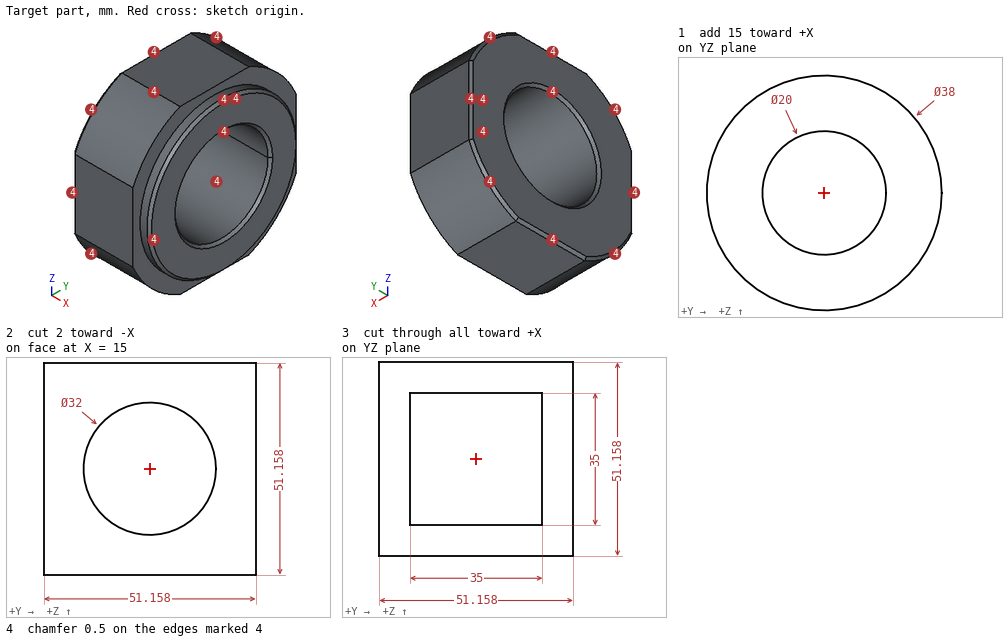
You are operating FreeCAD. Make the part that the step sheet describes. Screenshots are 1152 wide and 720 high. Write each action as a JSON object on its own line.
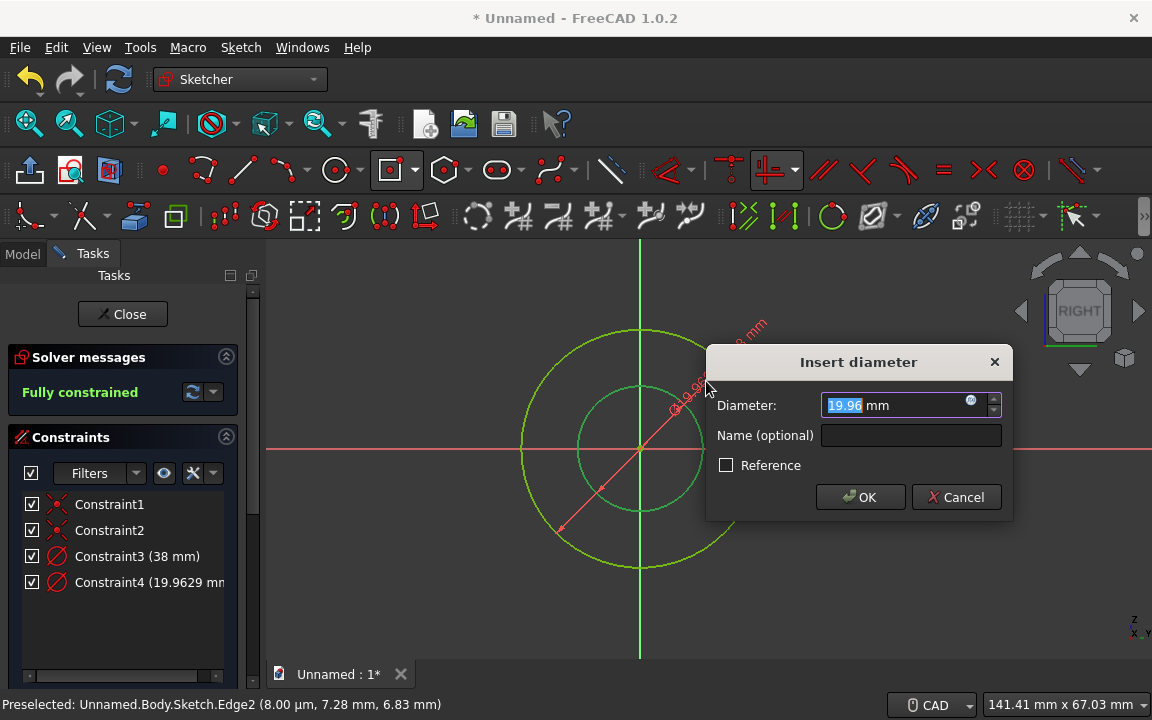
{"action": "type", "text": "20"}
{"action": "key", "text": "Return"}
{"action": "key", "text": "Escape"}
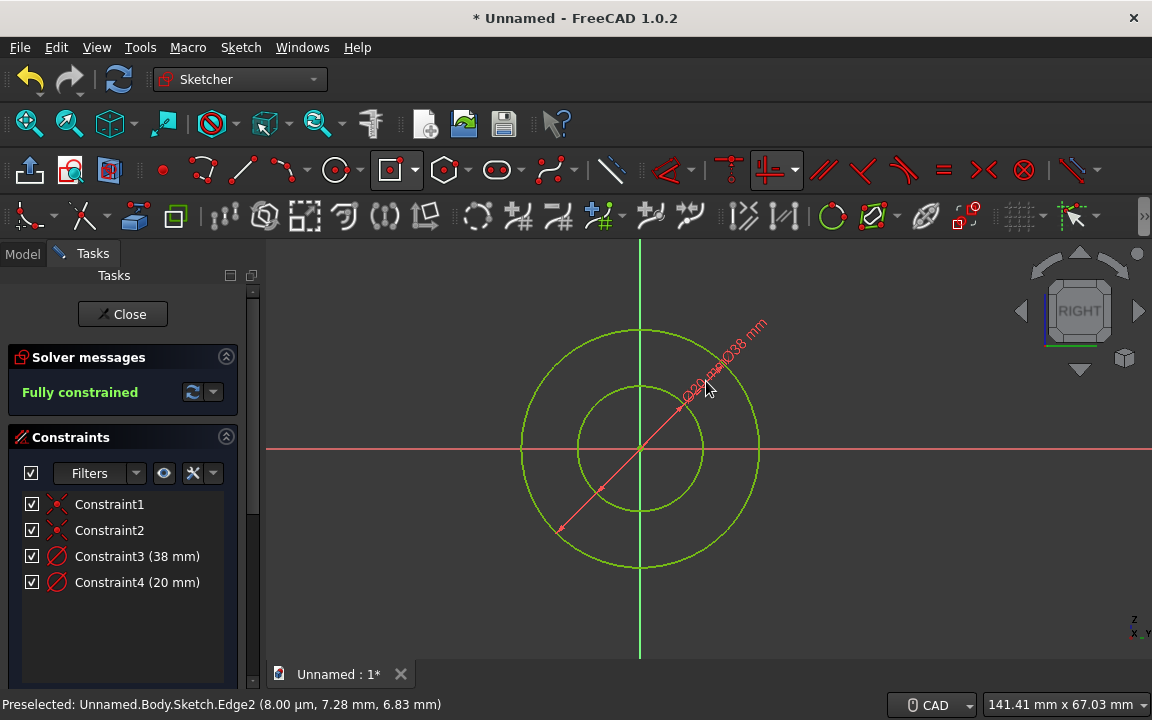
{"action": "left_click", "coordinate": [123, 314]}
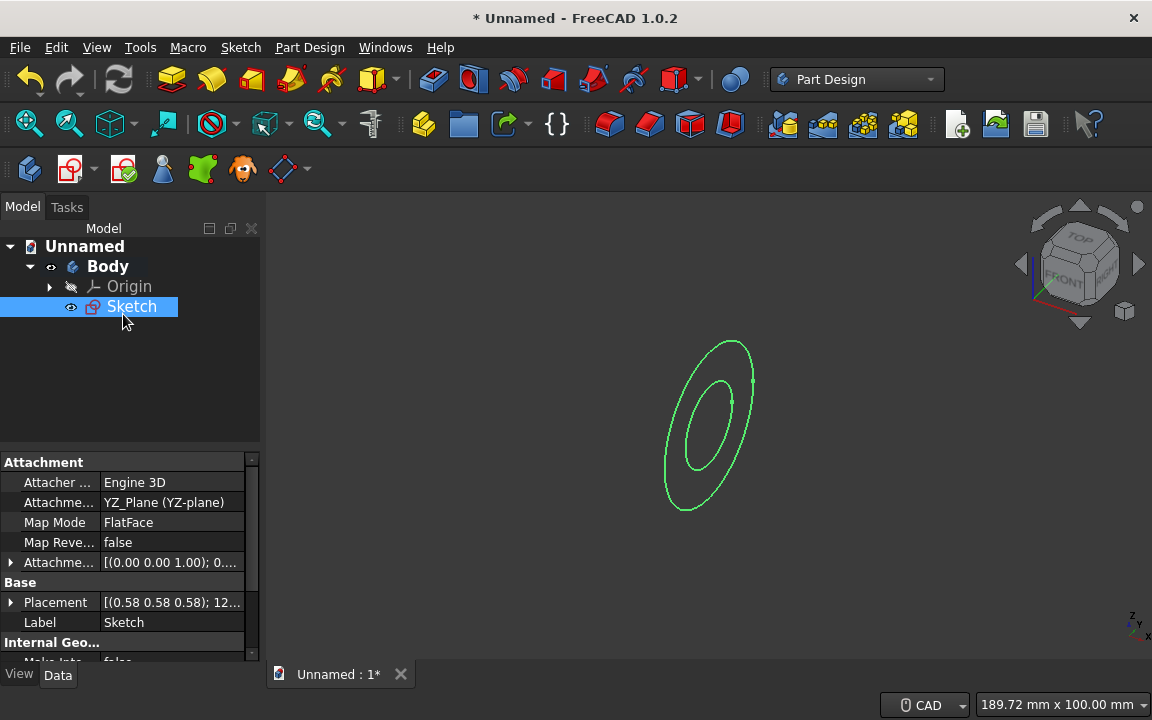
{"action": "left_click", "coordinate": [172, 80]}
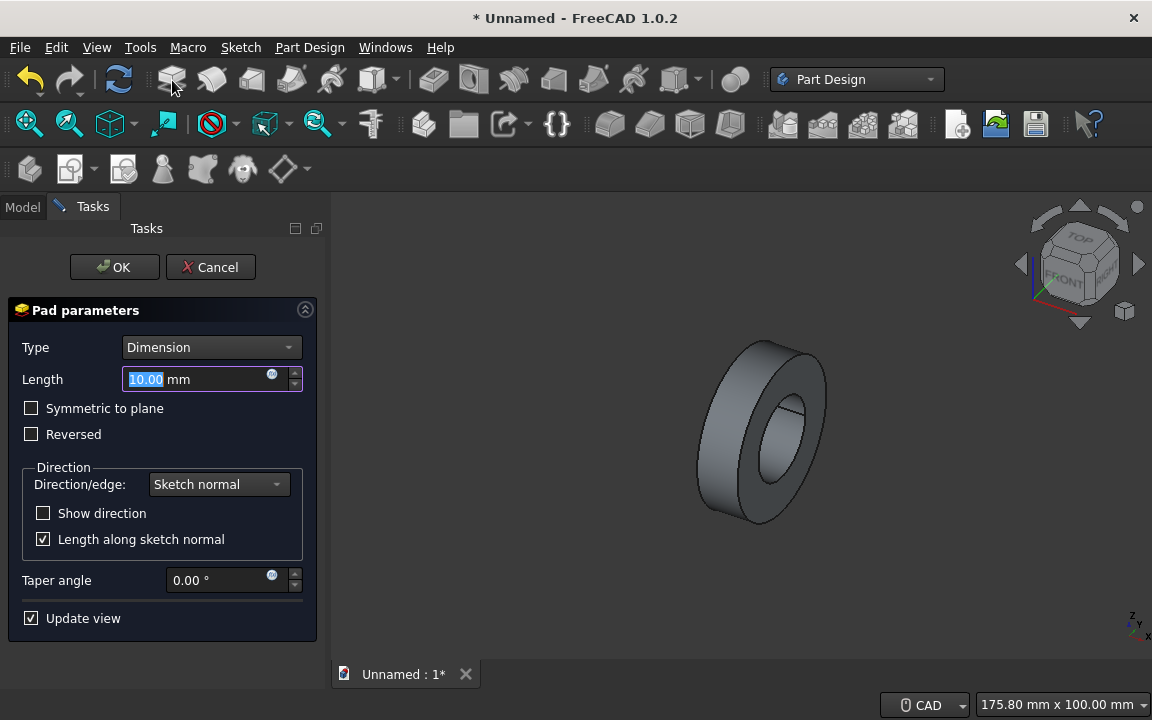
{"action": "type", "text": "15"}
{"action": "key", "text": "Tab"}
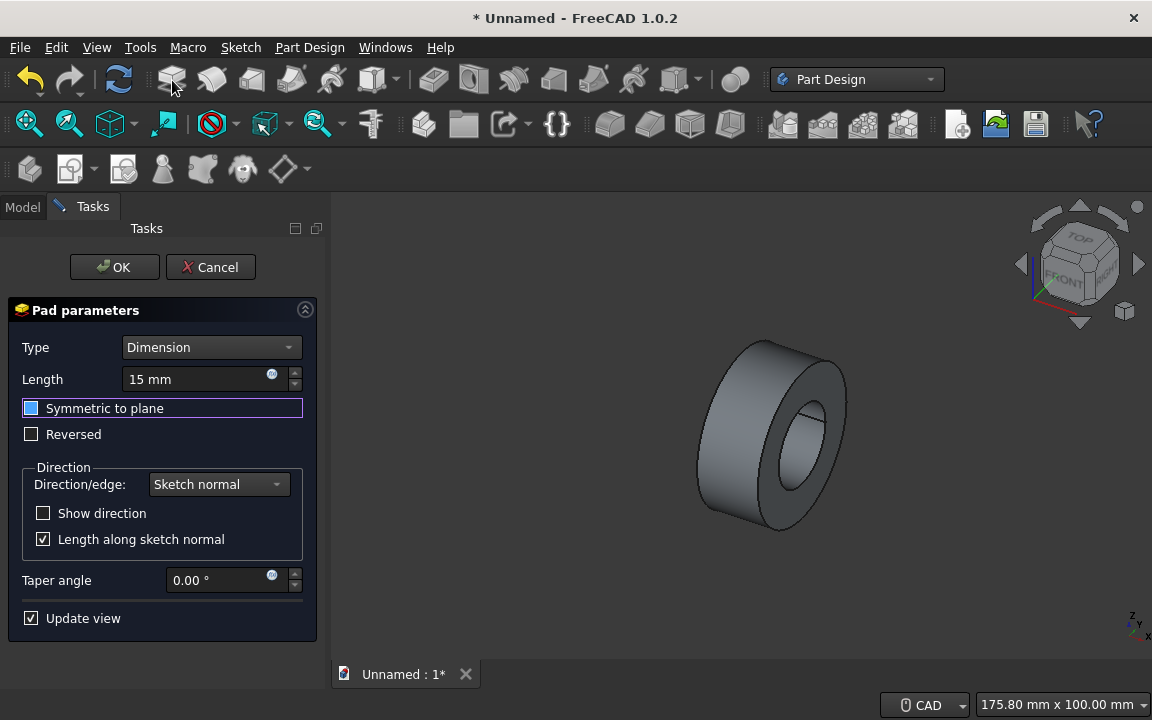
{"action": "left_click", "coordinate": [115, 267]}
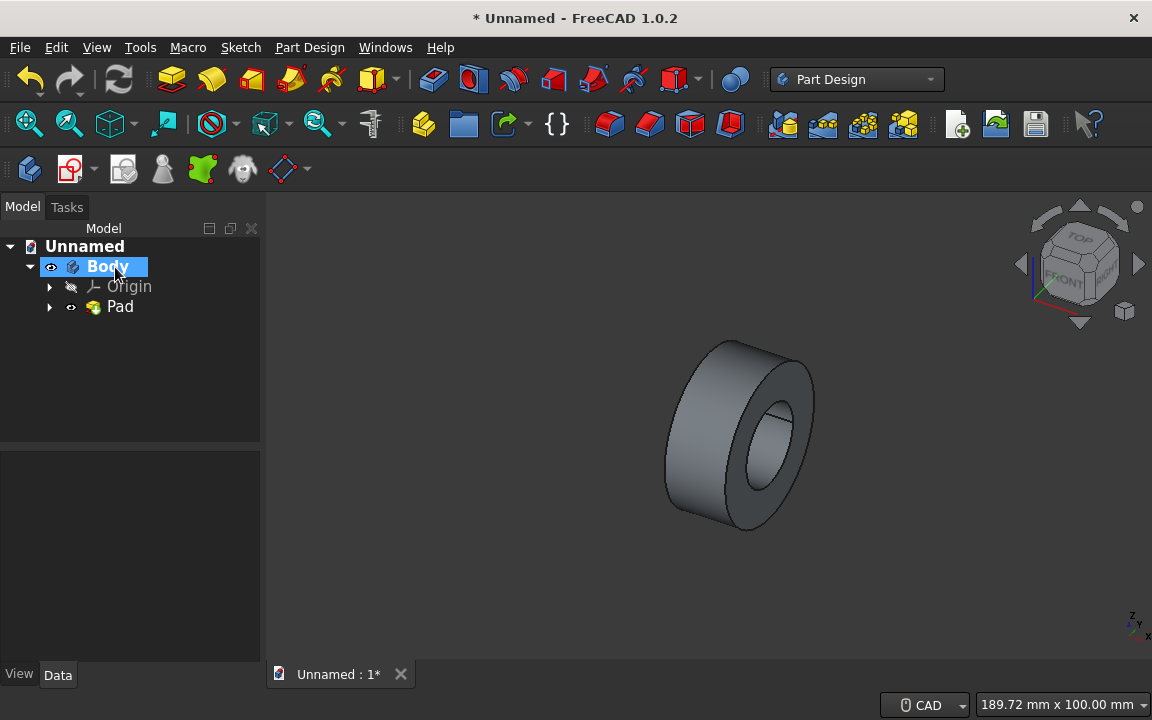
{"action": "left_click", "coordinate": [795, 461]}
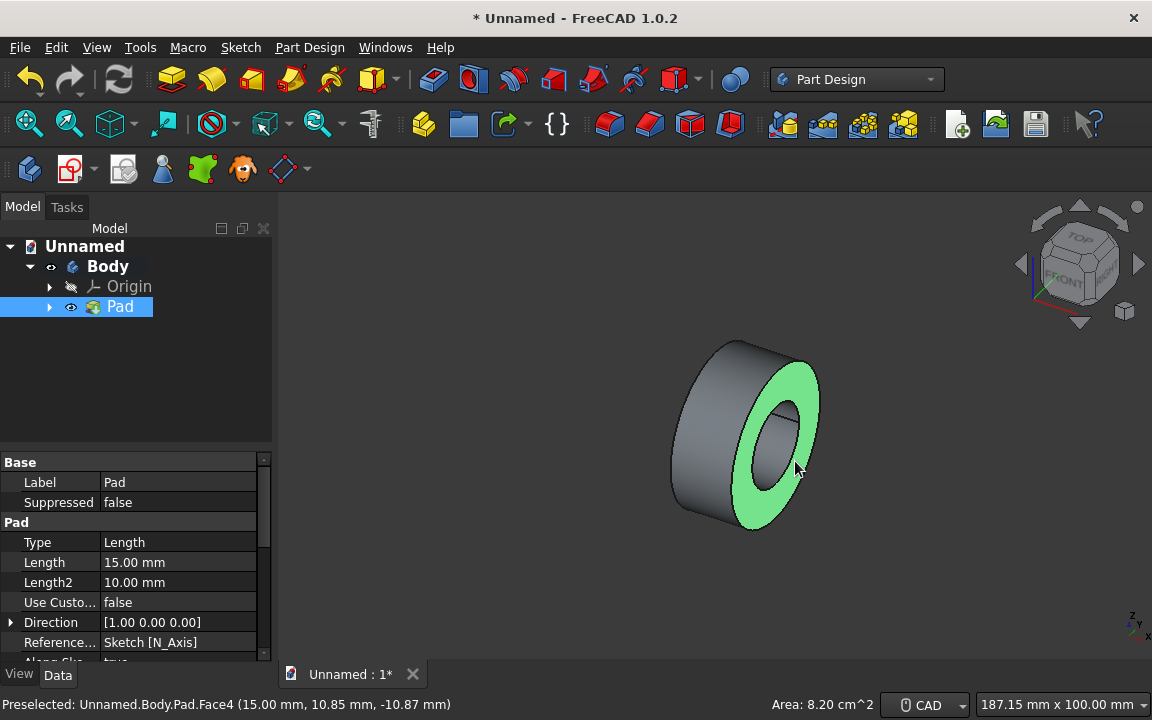
{"action": "left_click", "coordinate": [70, 170]}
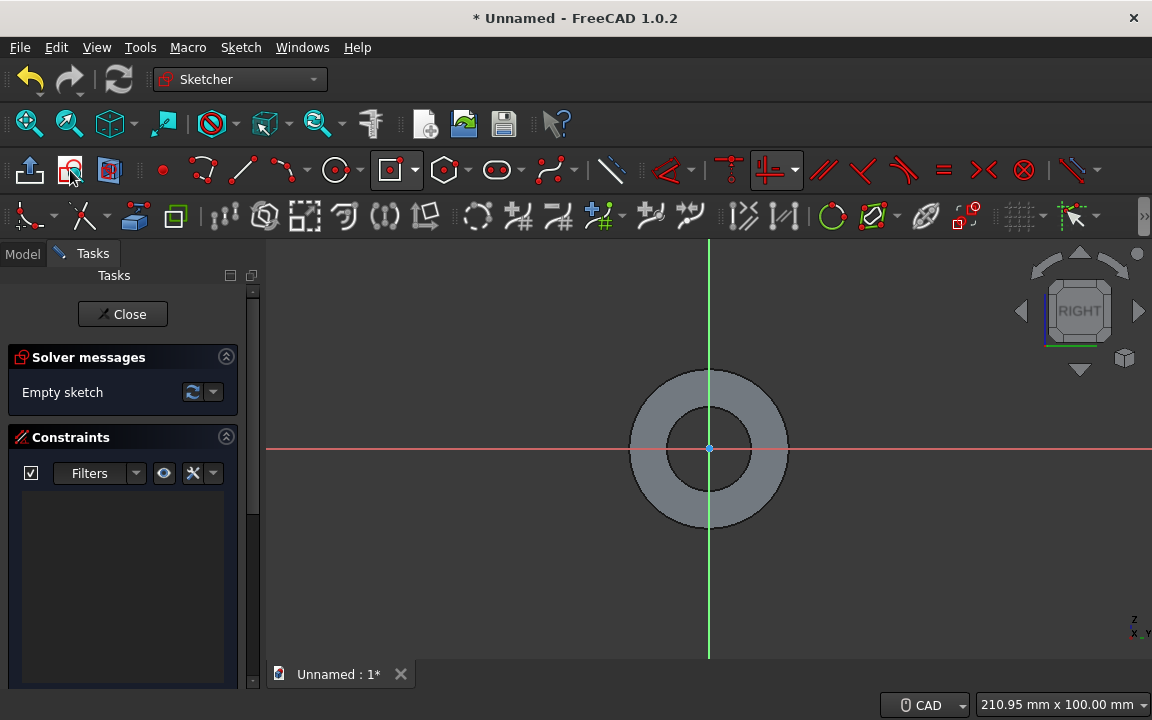
{"action": "key", "text": "g v"}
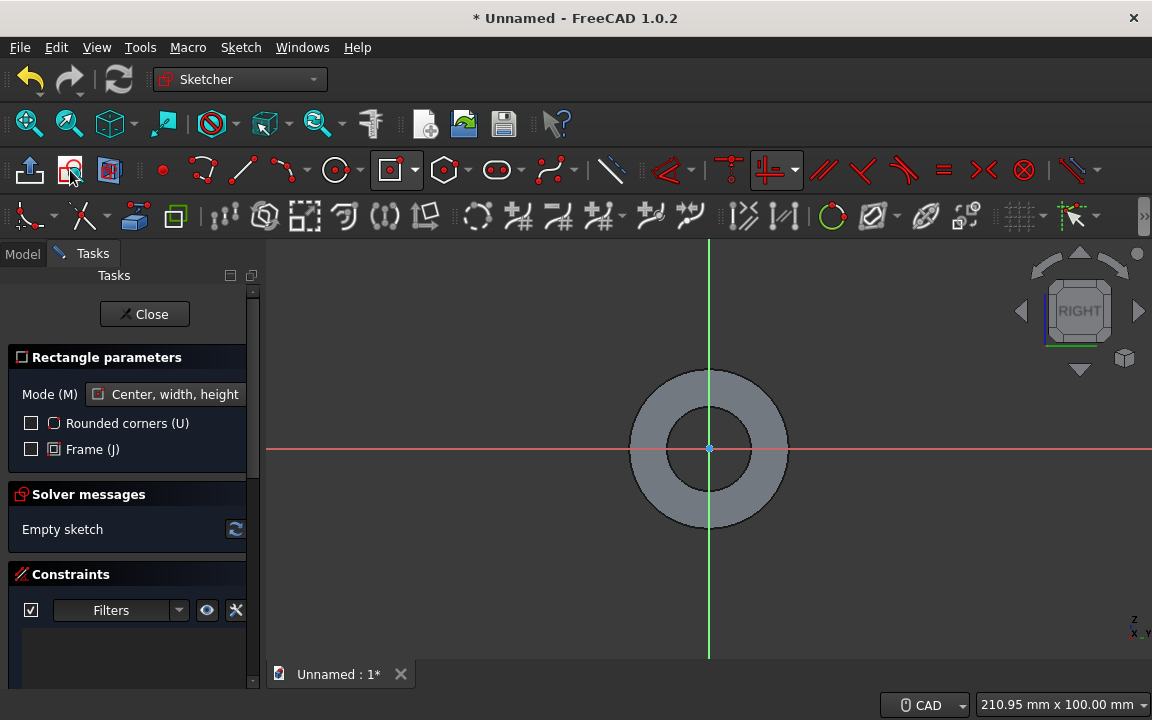
{"action": "left_click", "coordinate": [709, 449]}
{"action": "left_click", "coordinate": [816, 342]}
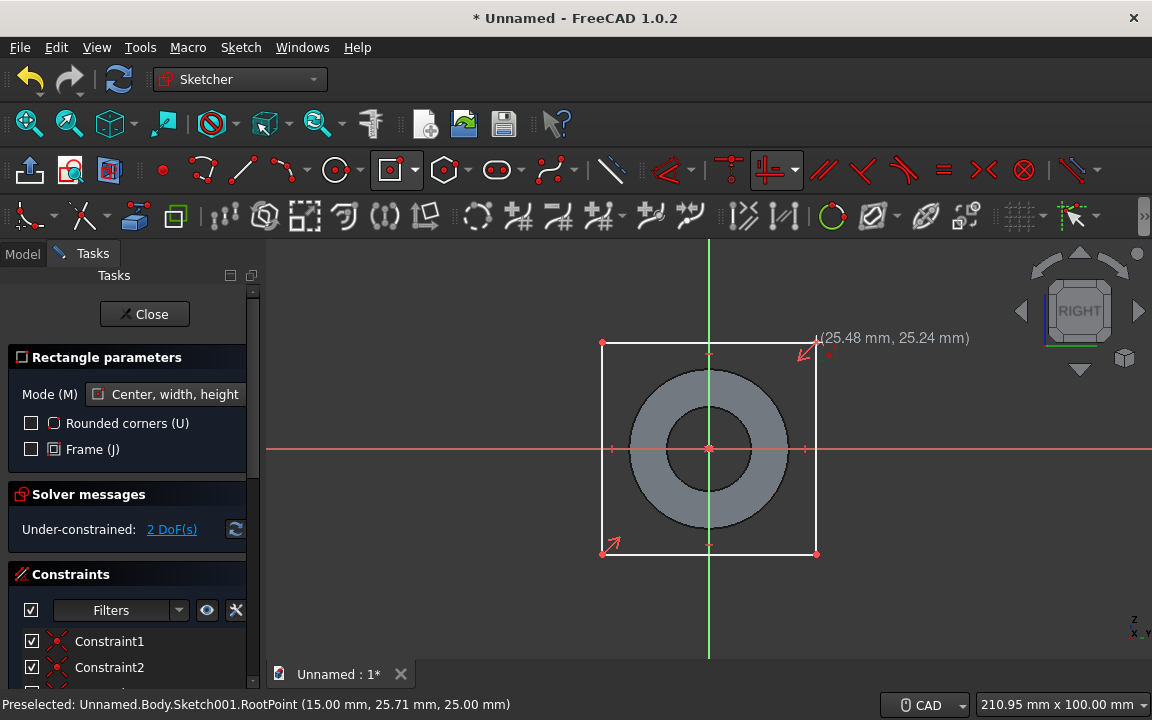
{"action": "key", "text": "g c"}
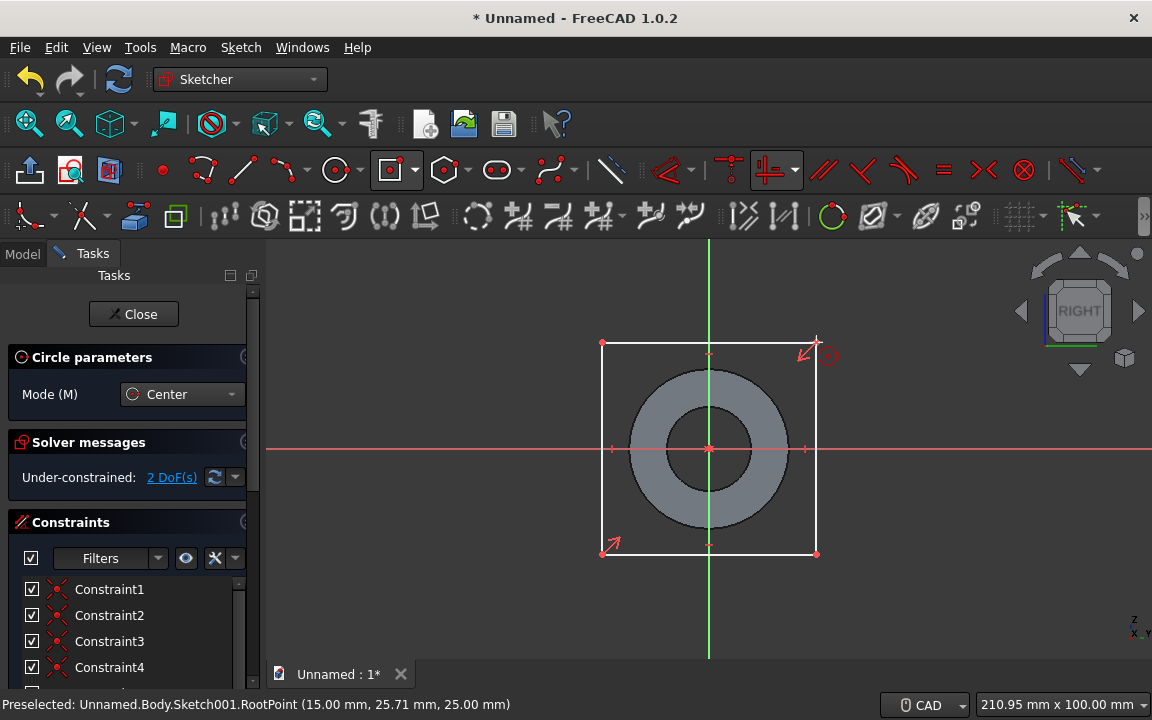
{"action": "left_click", "coordinate": [709, 449]}
{"action": "left_click", "coordinate": [757, 401]}
{"action": "key", "text": "Escape"}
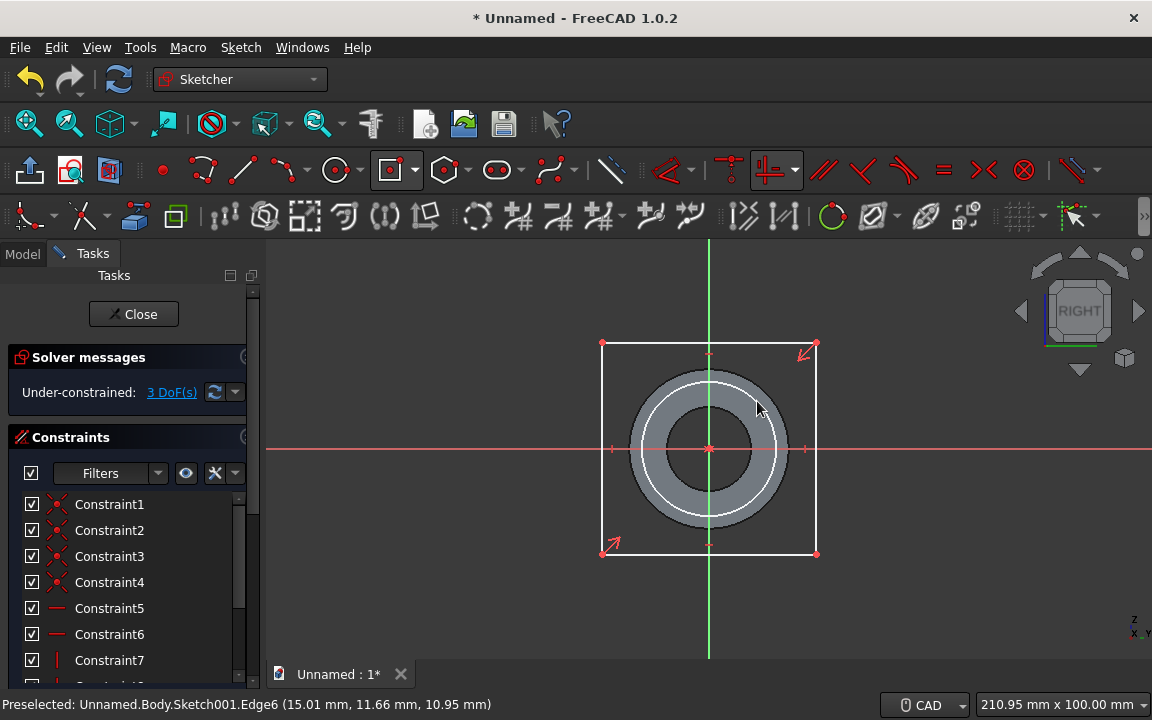
{"action": "key", "text": "d"}